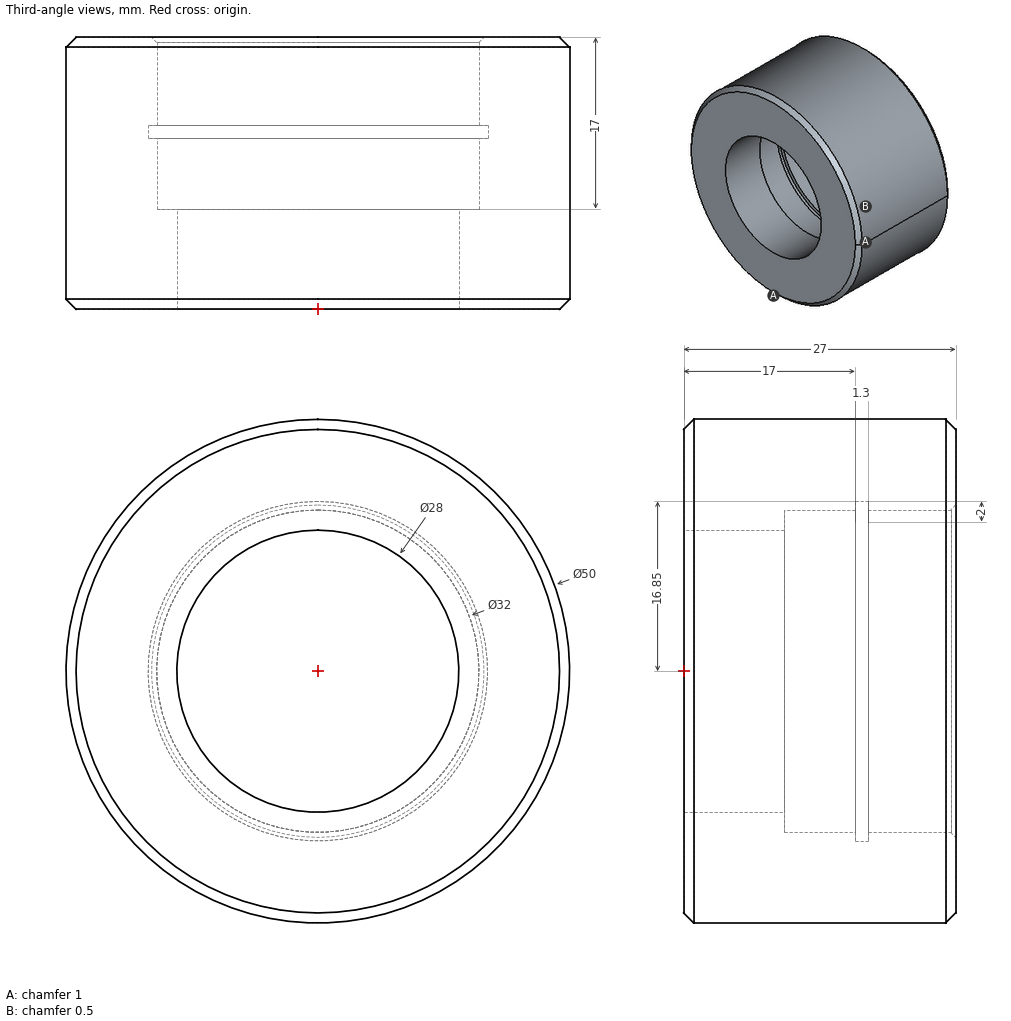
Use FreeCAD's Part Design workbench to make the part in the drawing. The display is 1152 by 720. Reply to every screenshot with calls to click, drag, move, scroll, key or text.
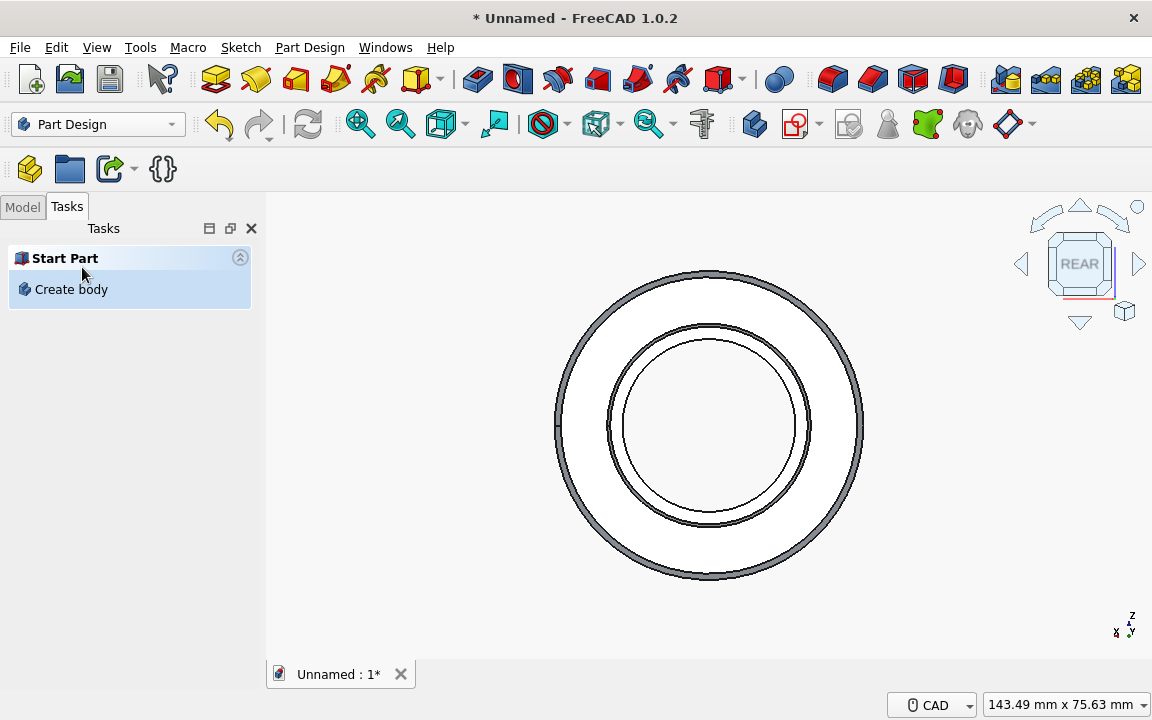
key(0)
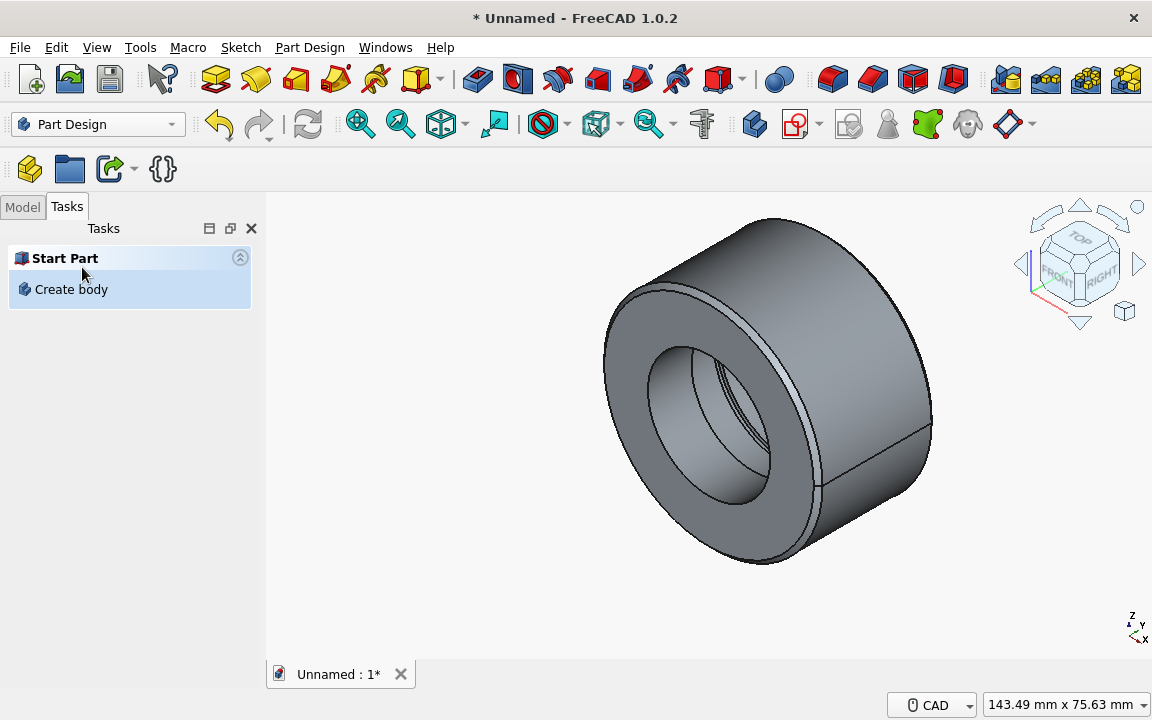
click(362, 124)